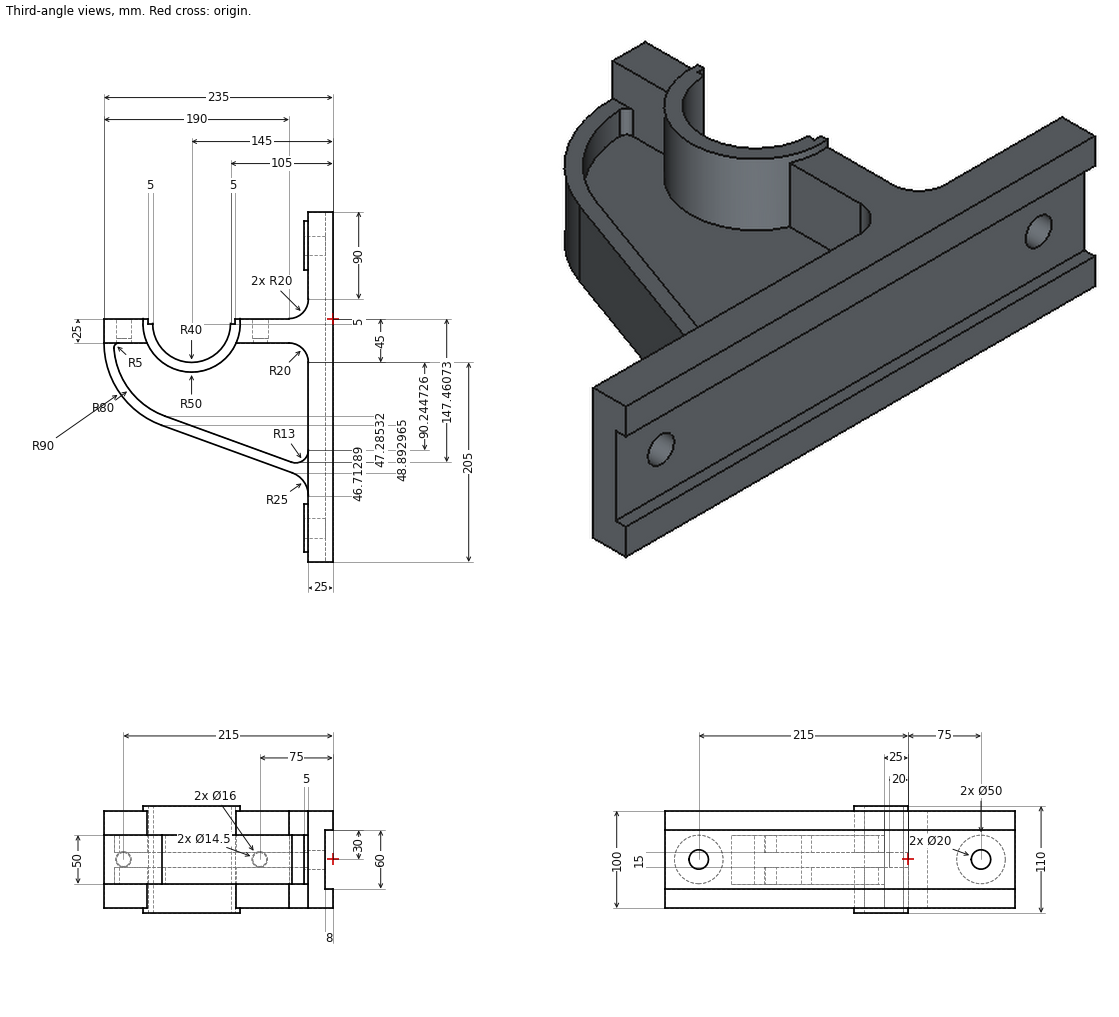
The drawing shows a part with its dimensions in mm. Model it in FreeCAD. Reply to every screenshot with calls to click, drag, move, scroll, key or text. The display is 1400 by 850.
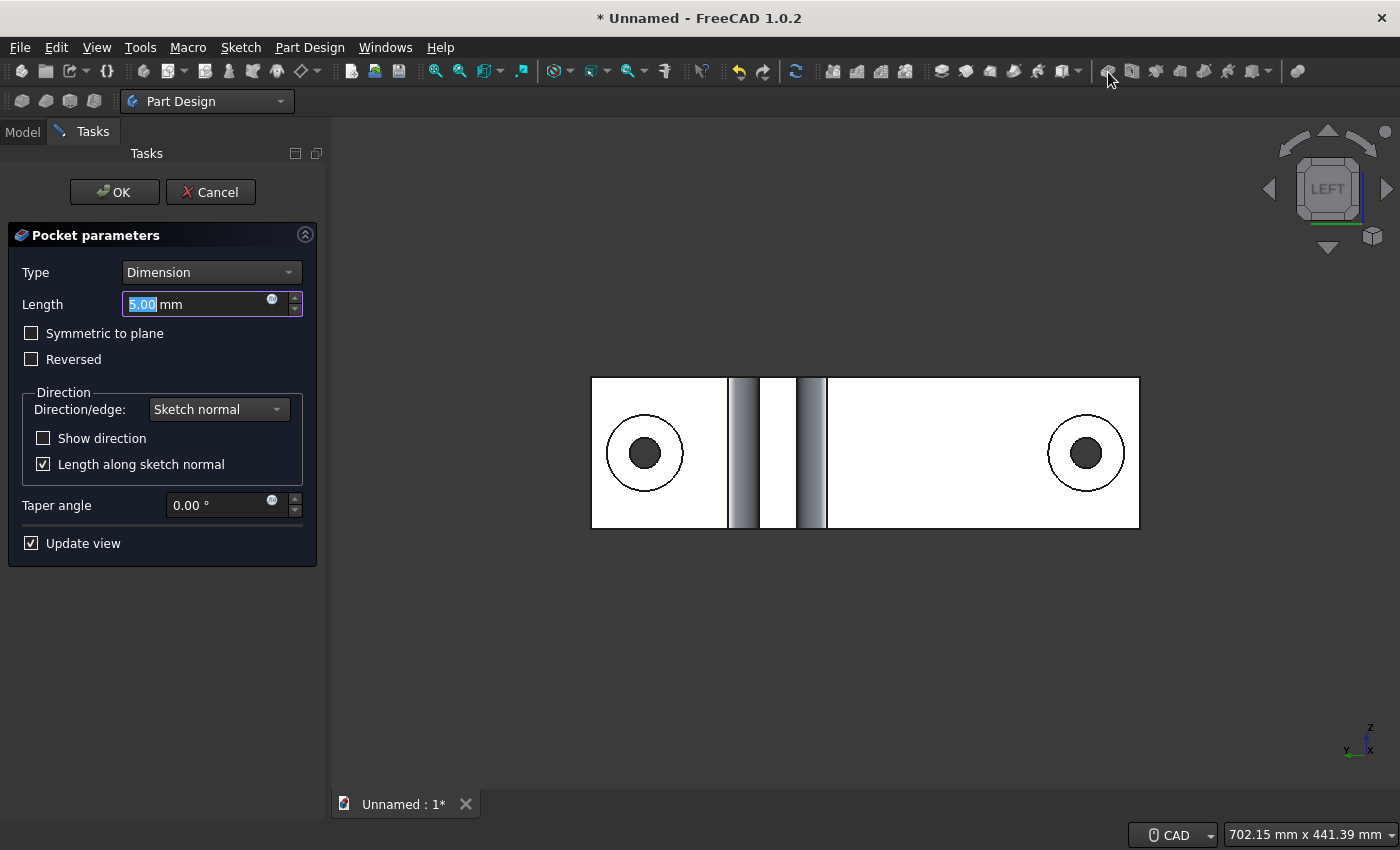
text(25)
key(Tab)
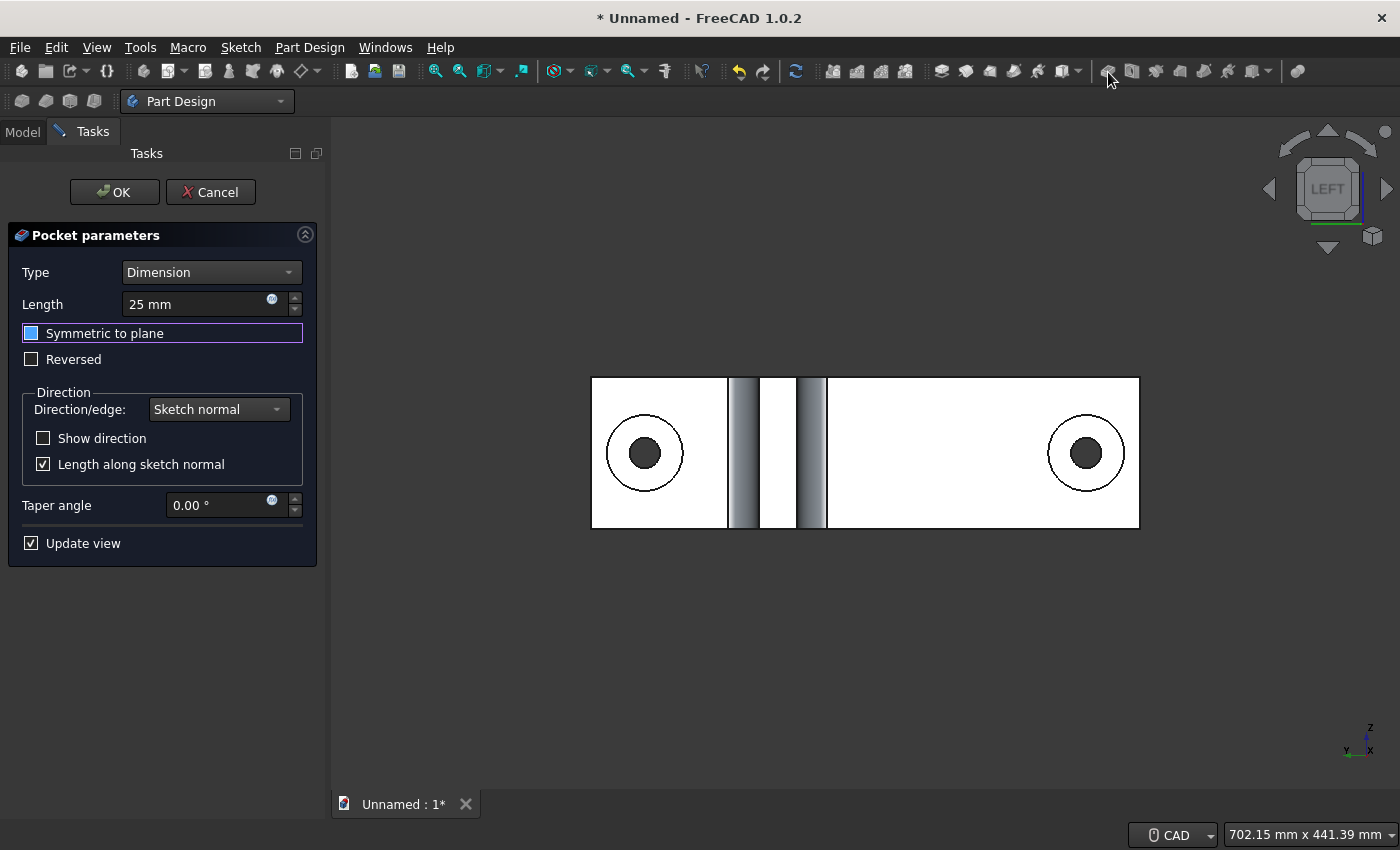
click(30, 359)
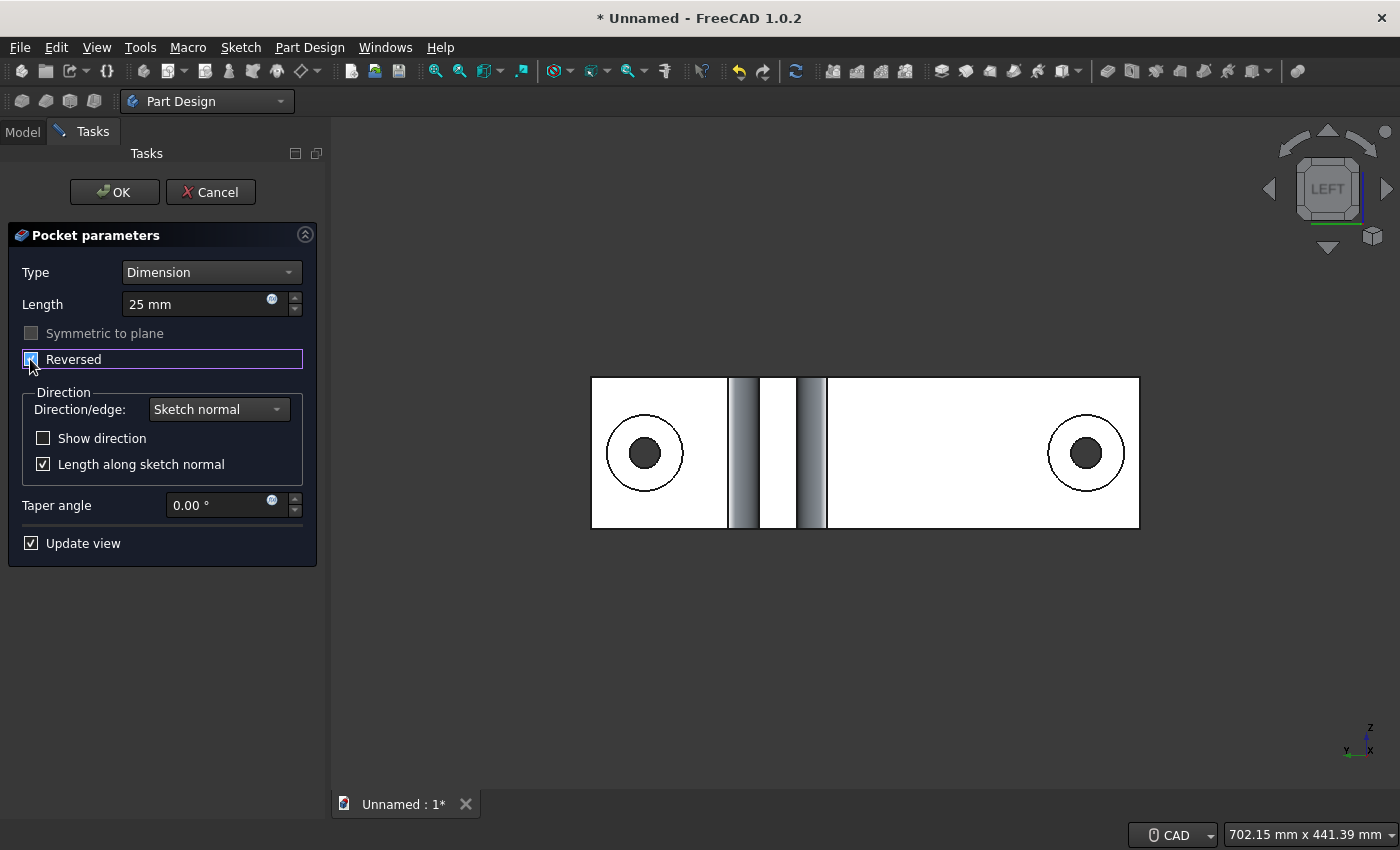
click(115, 192)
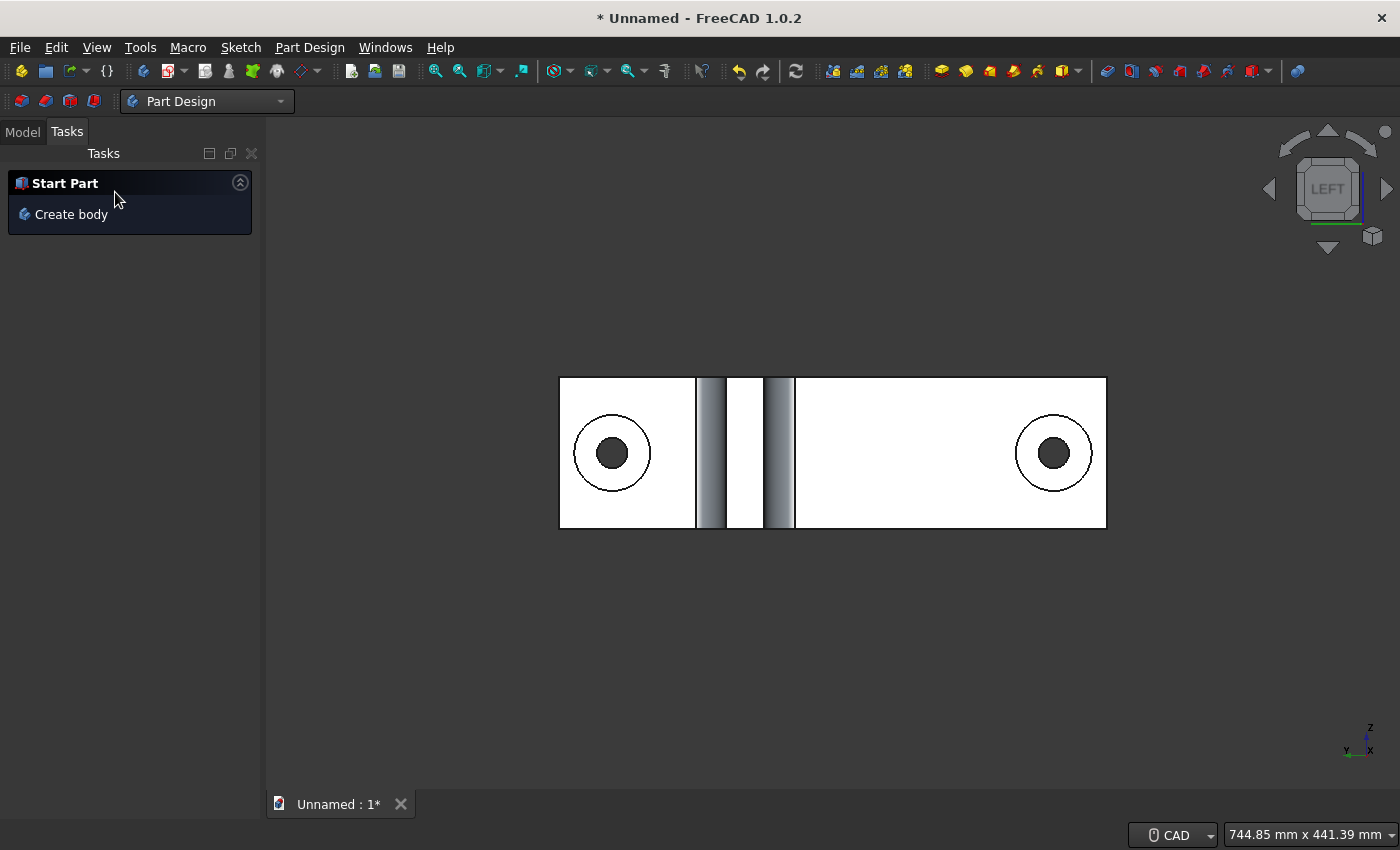
click(168, 72)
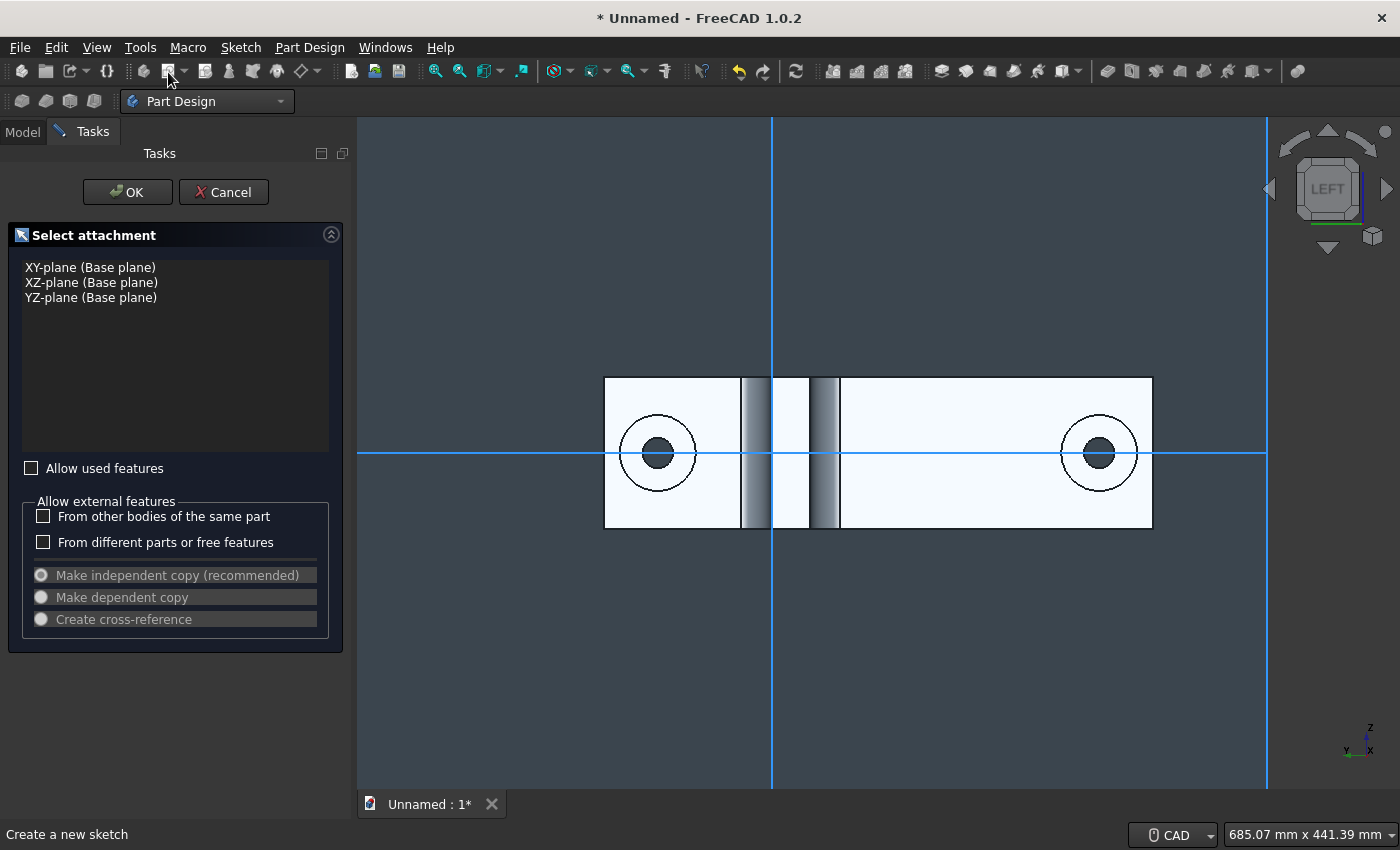
click(82, 282)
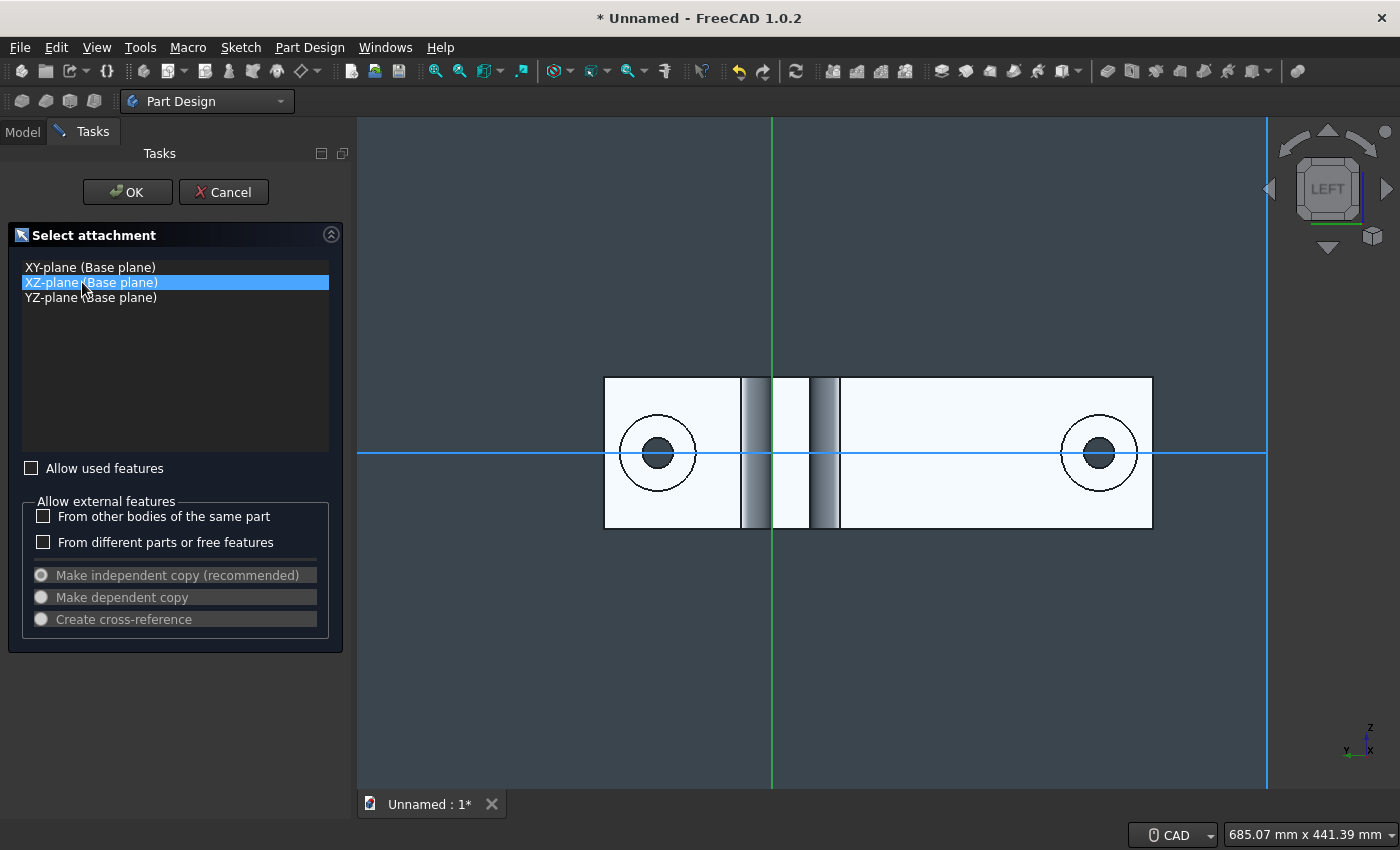
click(128, 192)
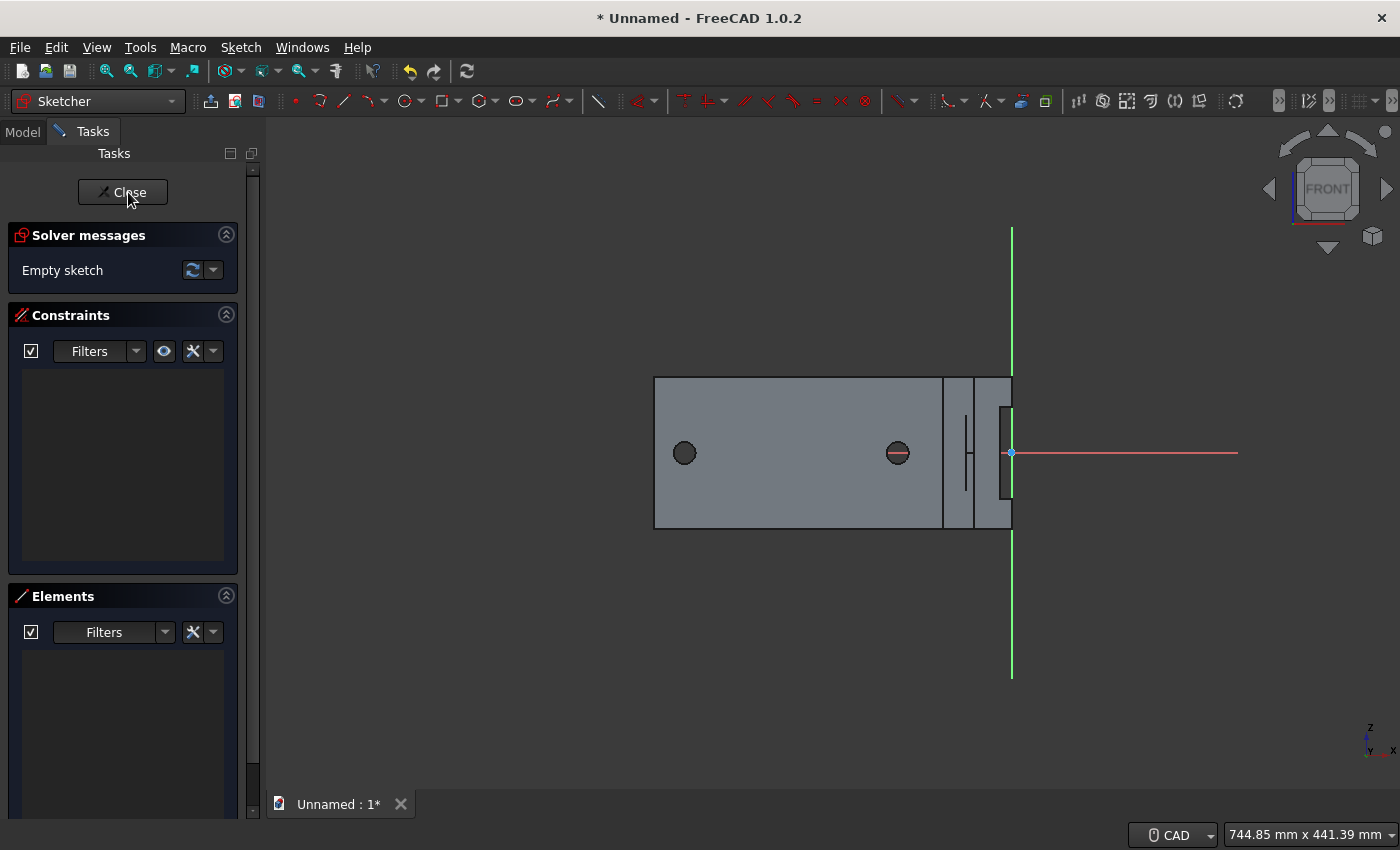
click(260, 102)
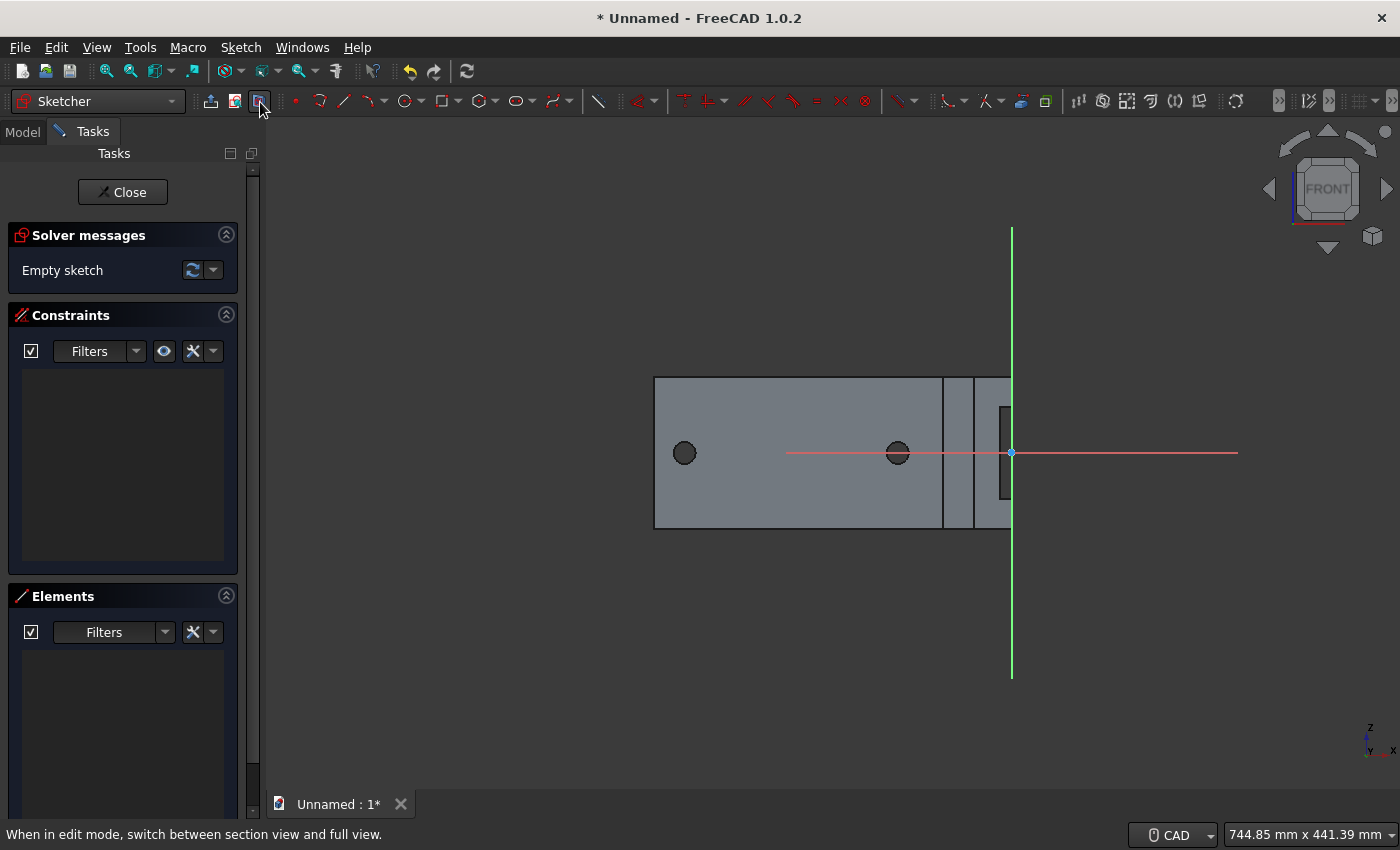
scroll(937, 453, up, 3)